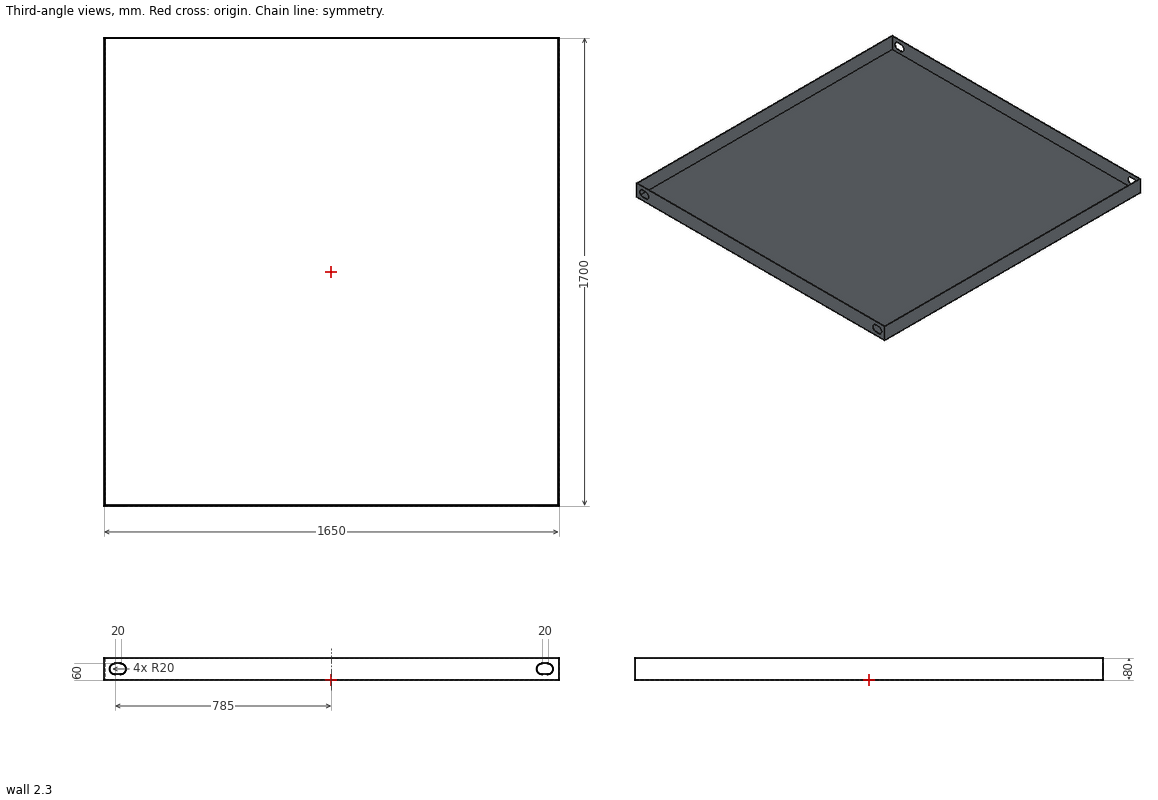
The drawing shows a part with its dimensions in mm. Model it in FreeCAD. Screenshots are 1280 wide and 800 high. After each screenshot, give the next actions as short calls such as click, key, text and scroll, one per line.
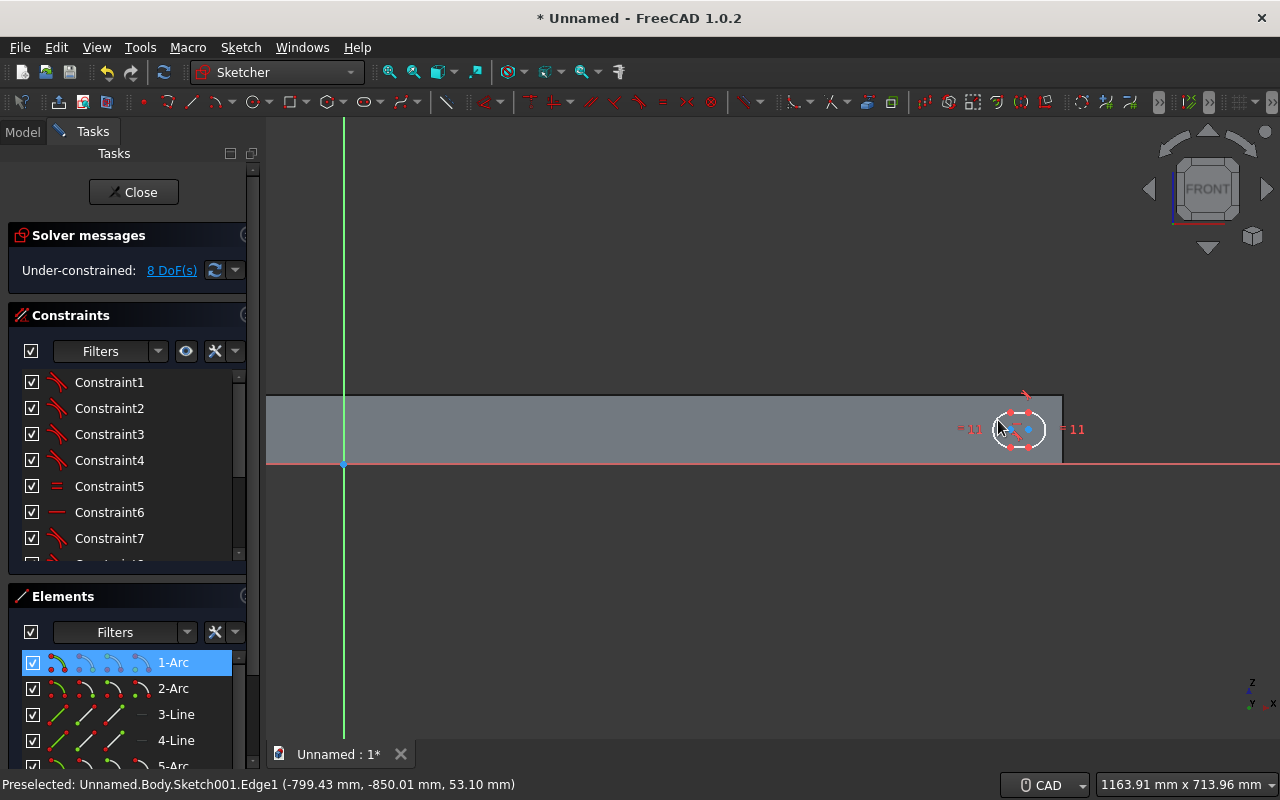
click(996, 420)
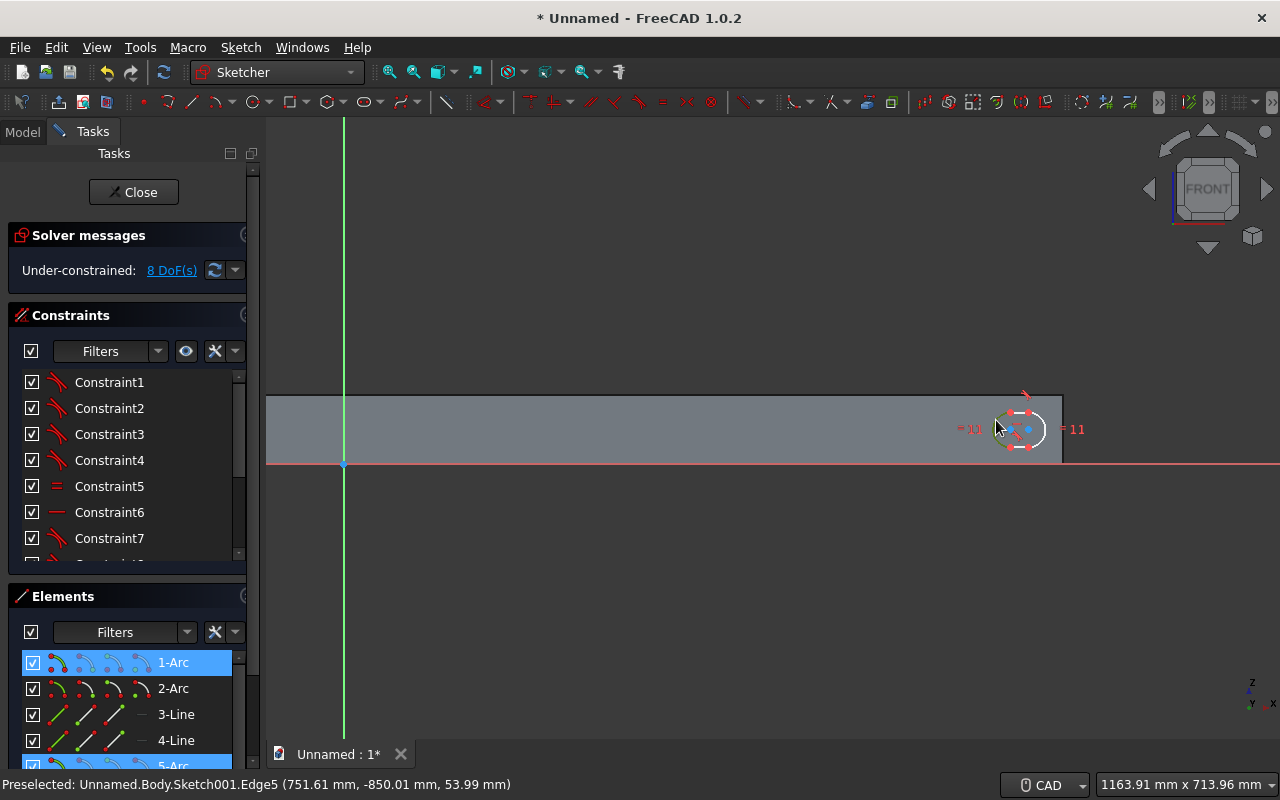
click(664, 102)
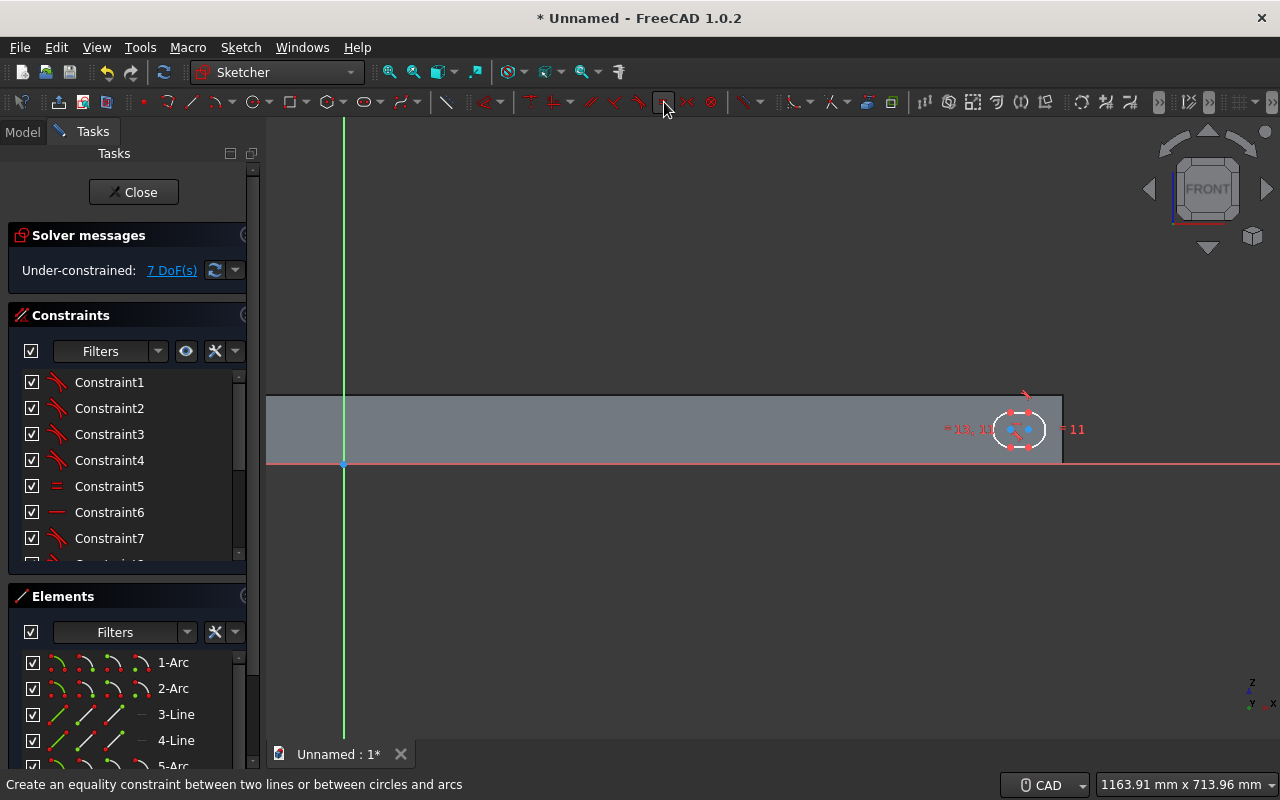
scroll(999, 420, down, 4)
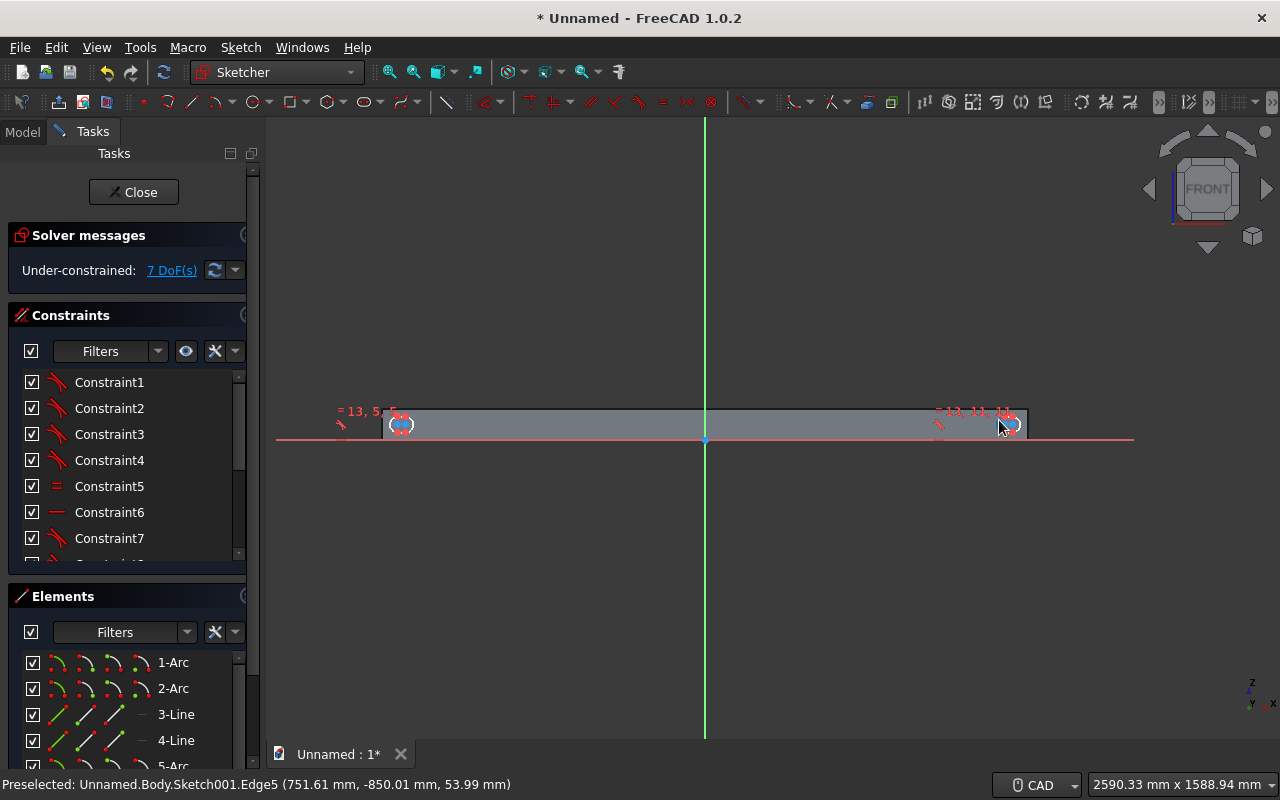
scroll(406, 425, up, 3)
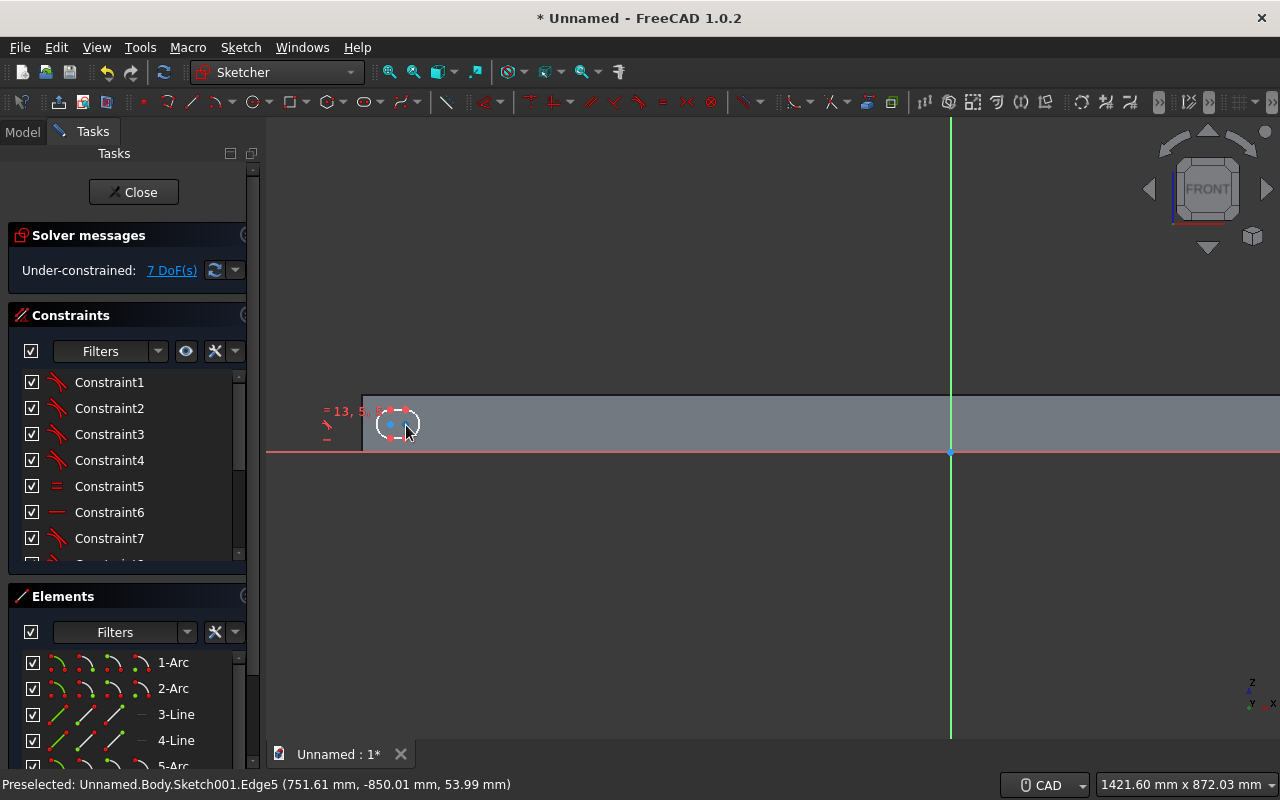
click(405, 424)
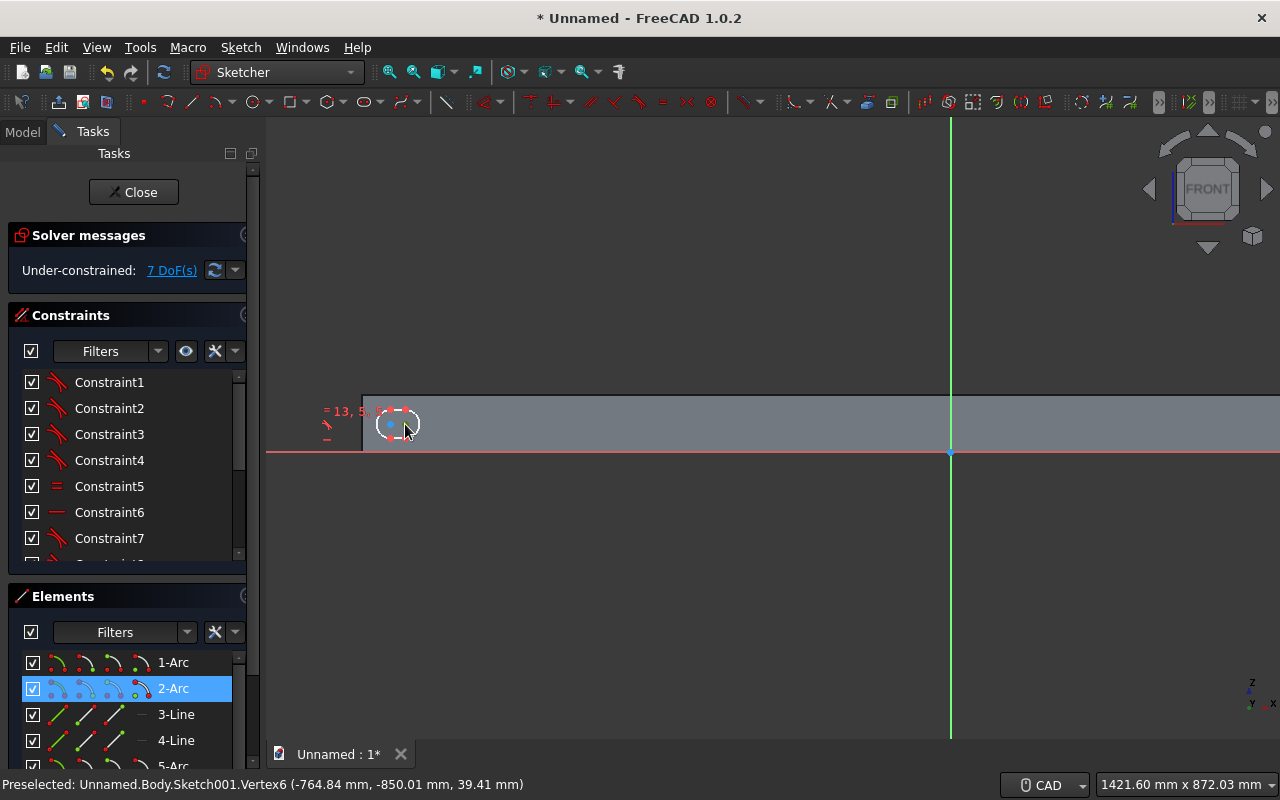
scroll(405, 425, down, 3)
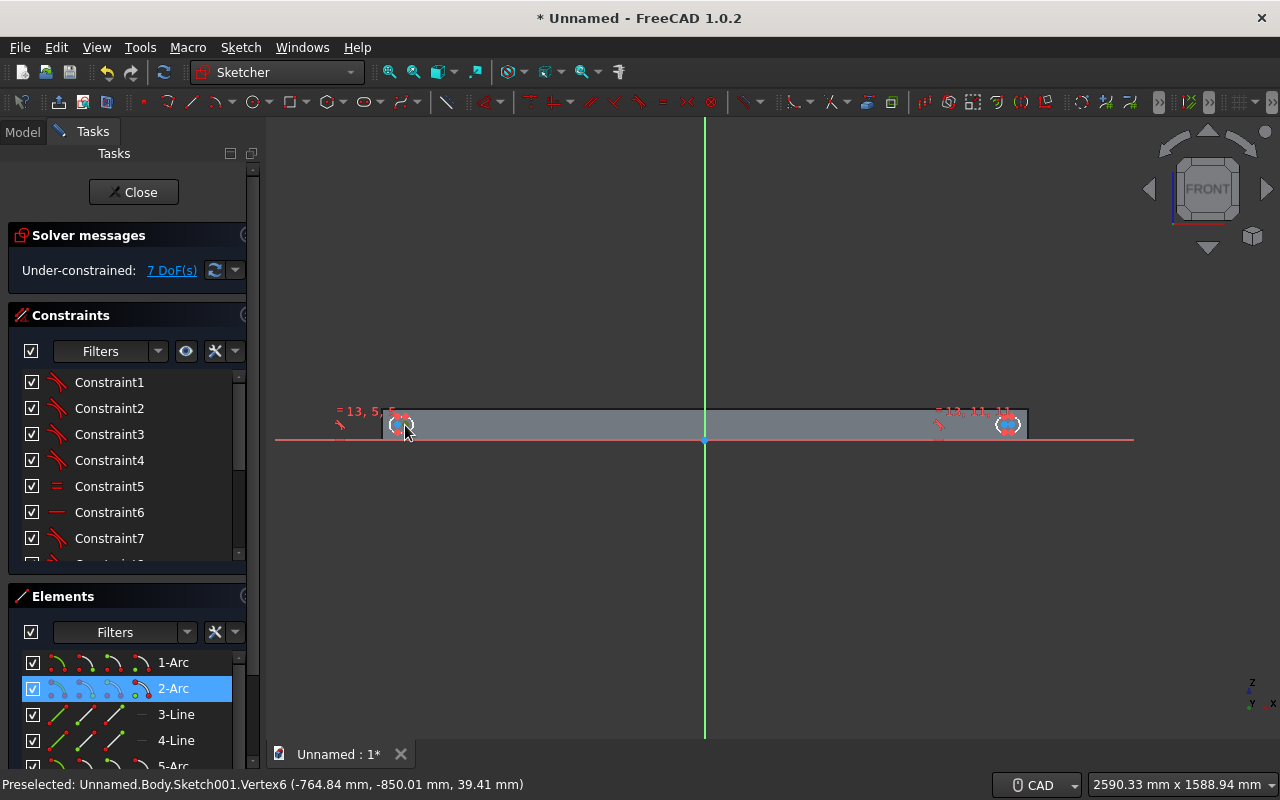
scroll(1004, 425, up, 3)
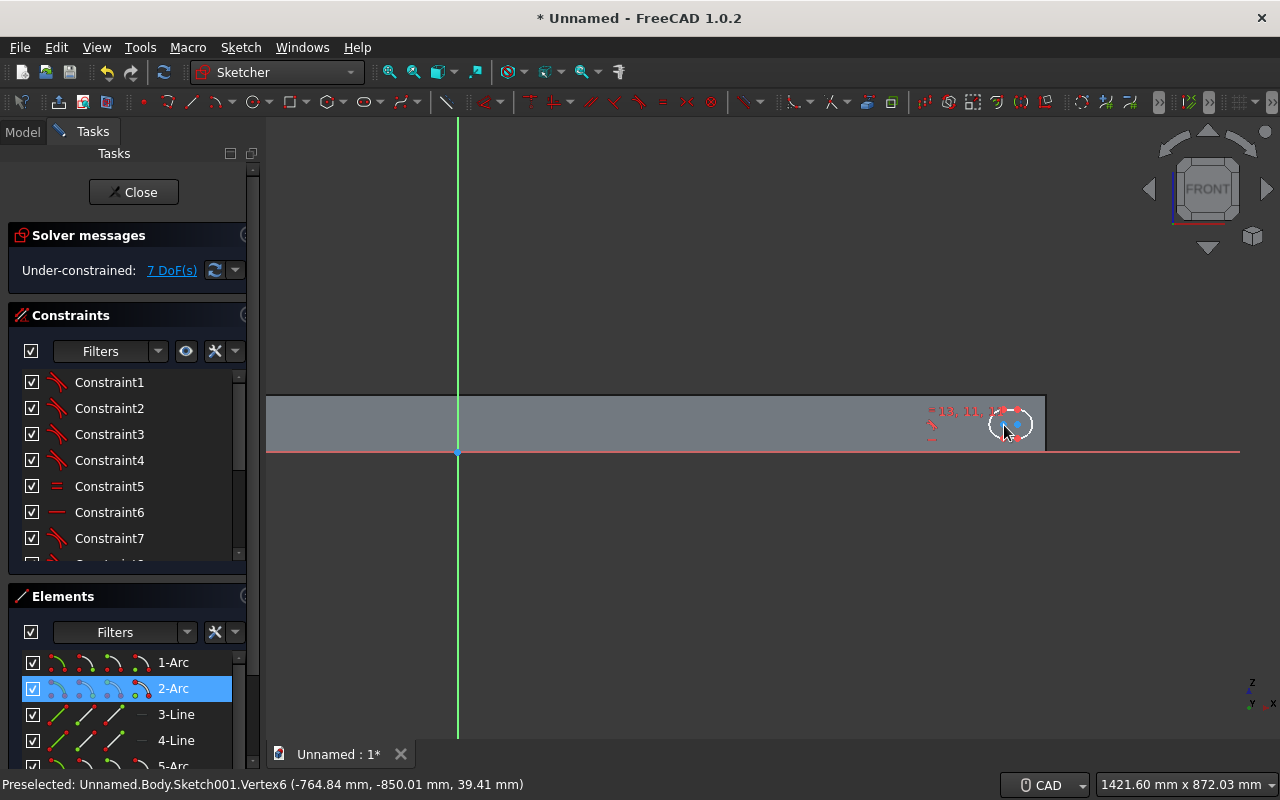
click(1004, 424)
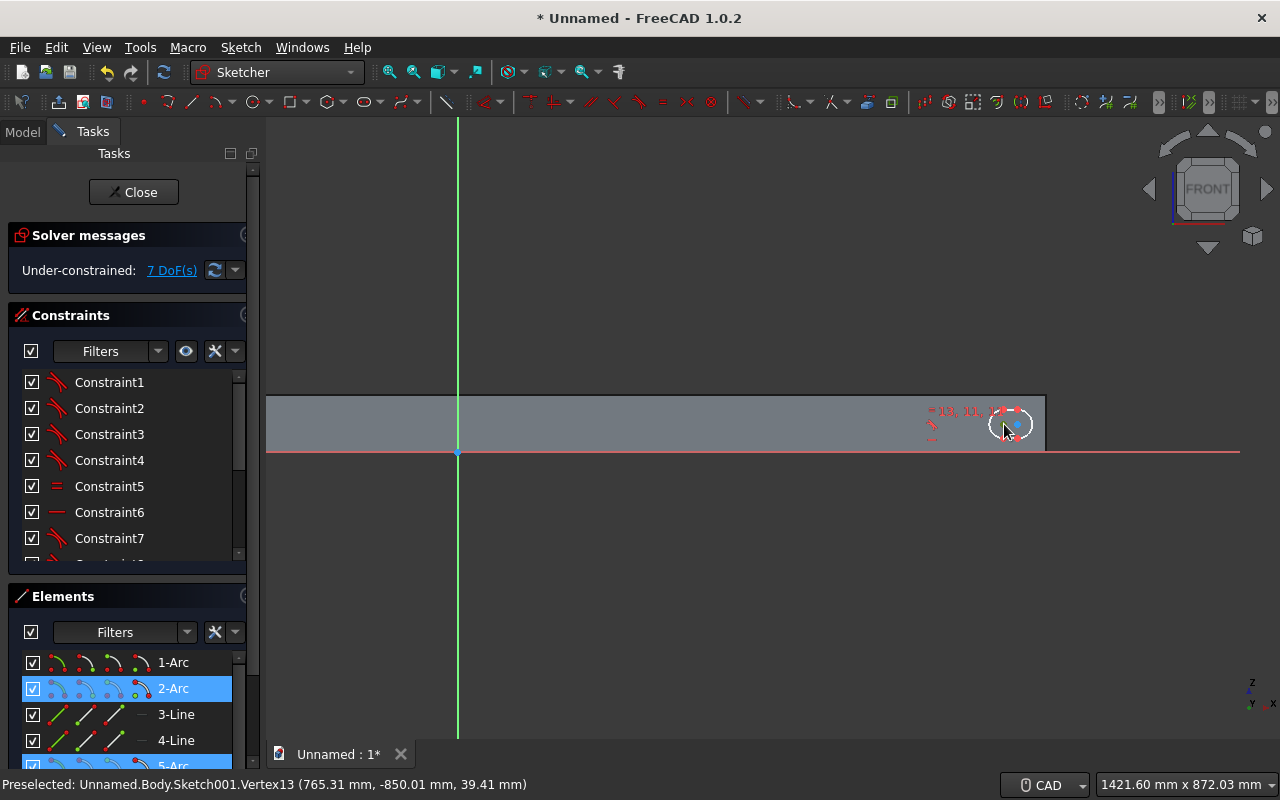
click(458, 671)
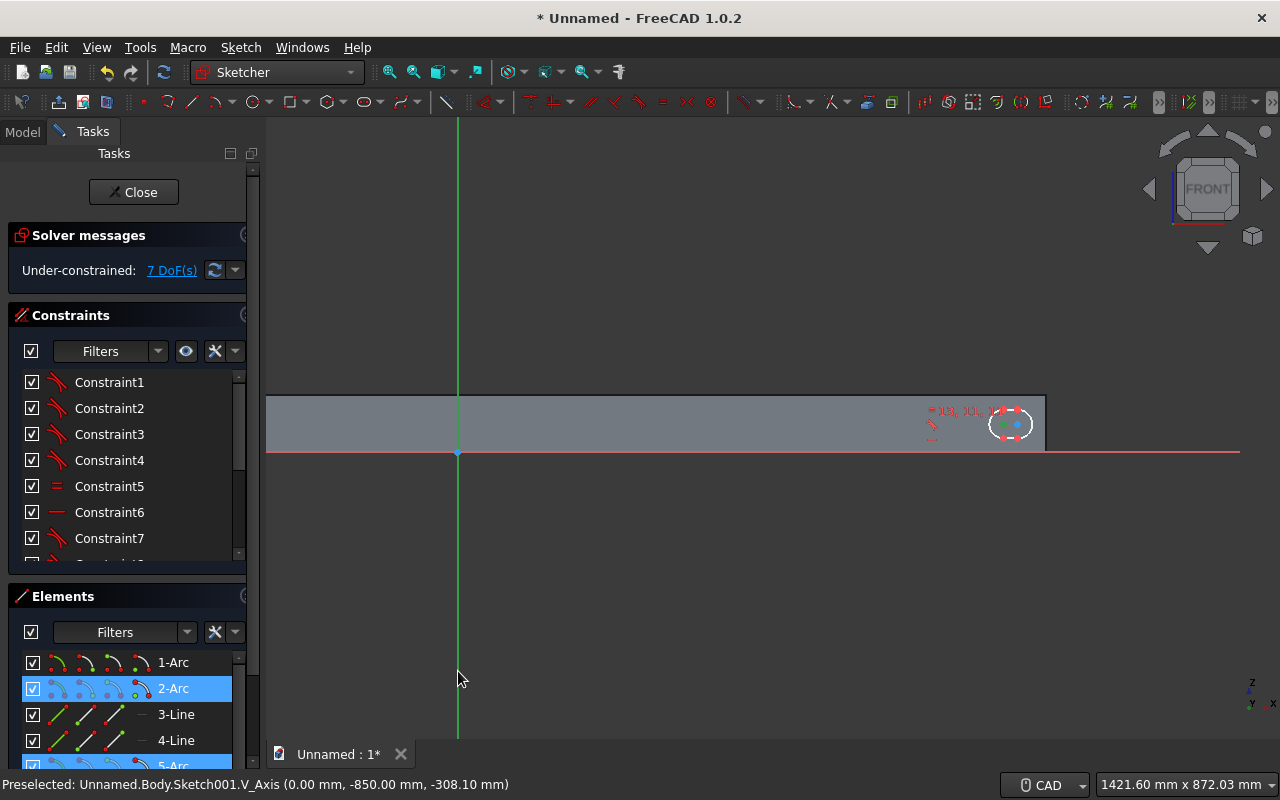
key(s)